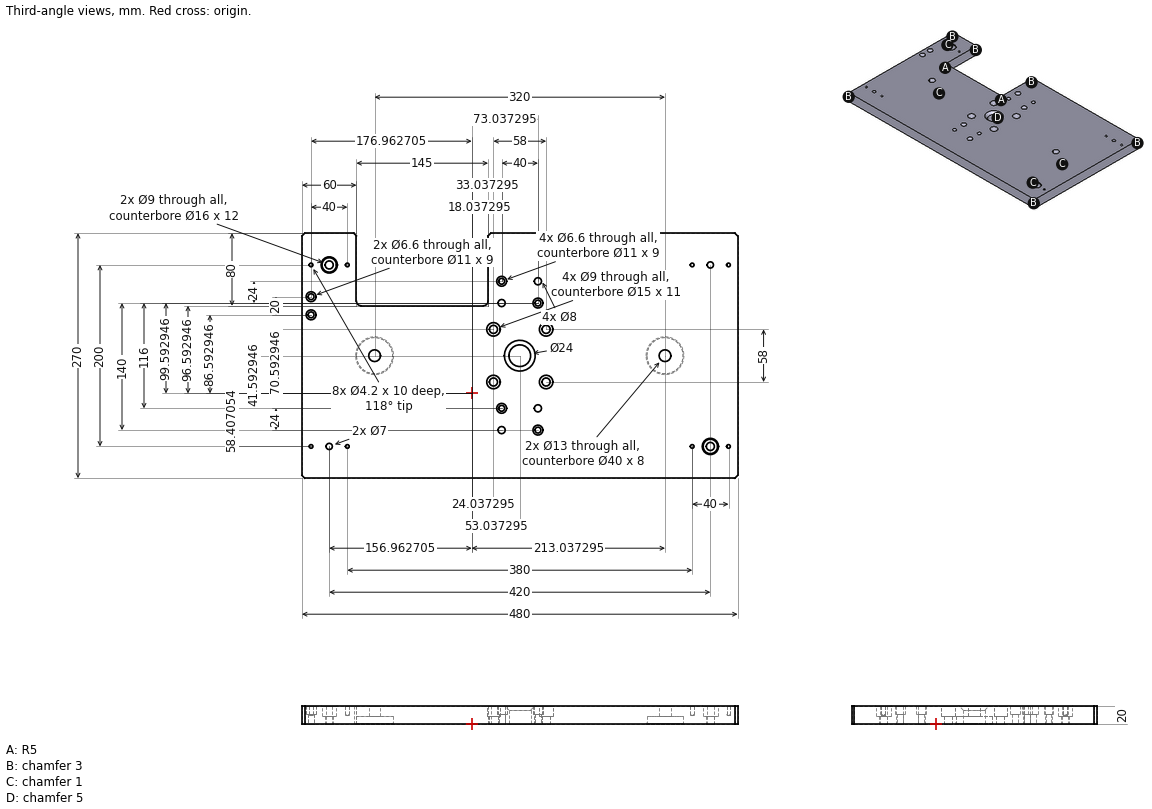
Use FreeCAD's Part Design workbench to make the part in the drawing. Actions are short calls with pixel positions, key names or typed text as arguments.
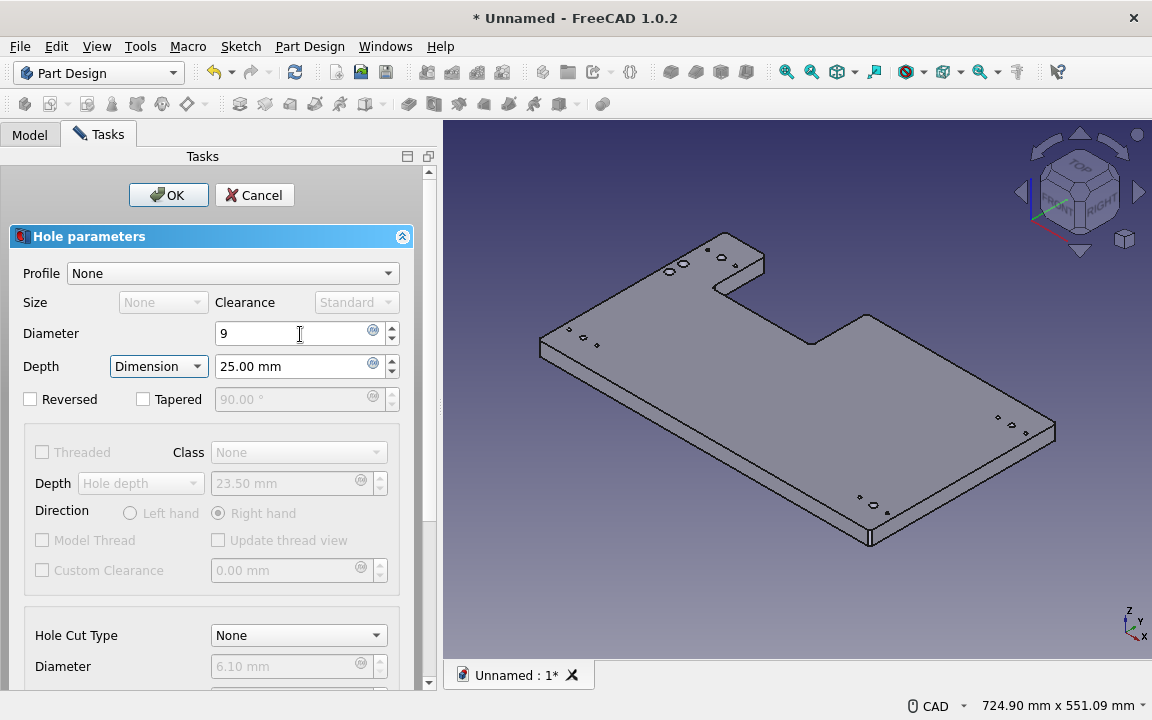
click(160, 366)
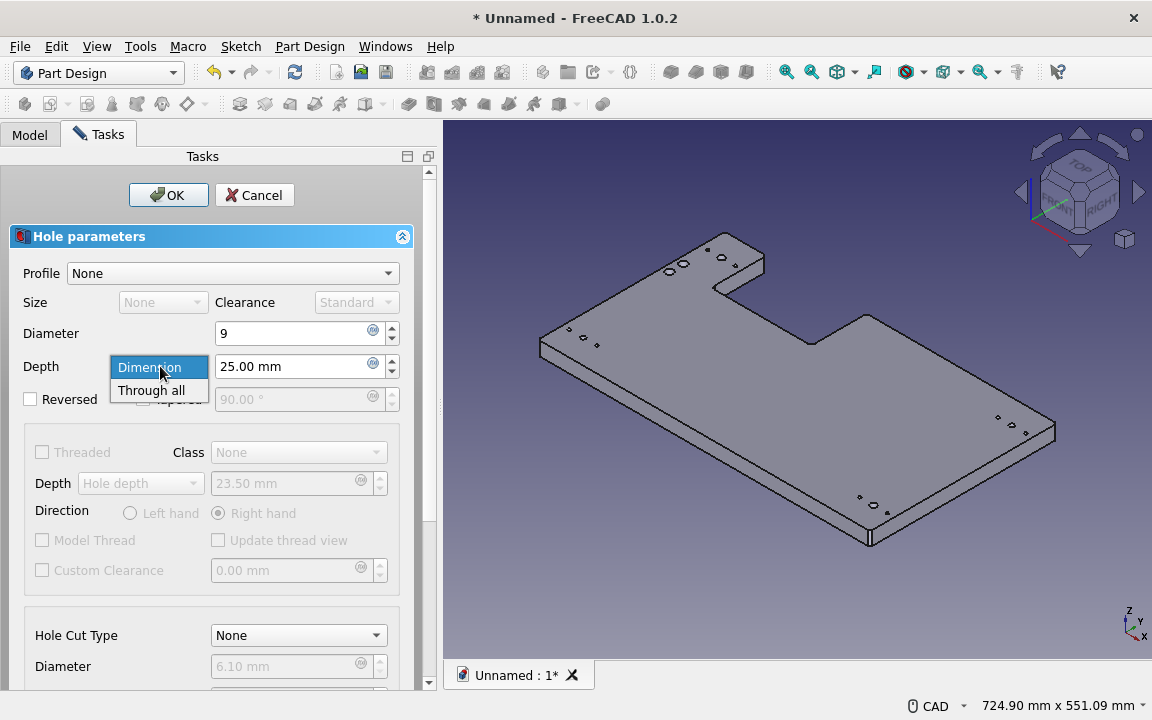
click(158, 390)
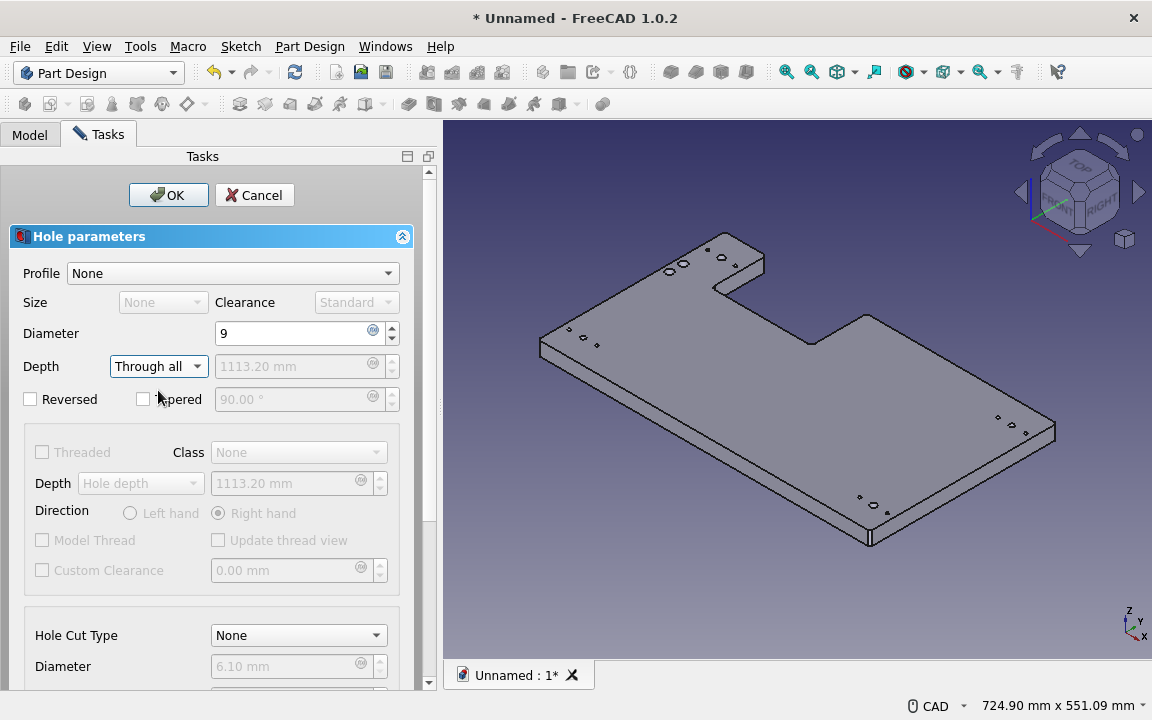
click(300, 636)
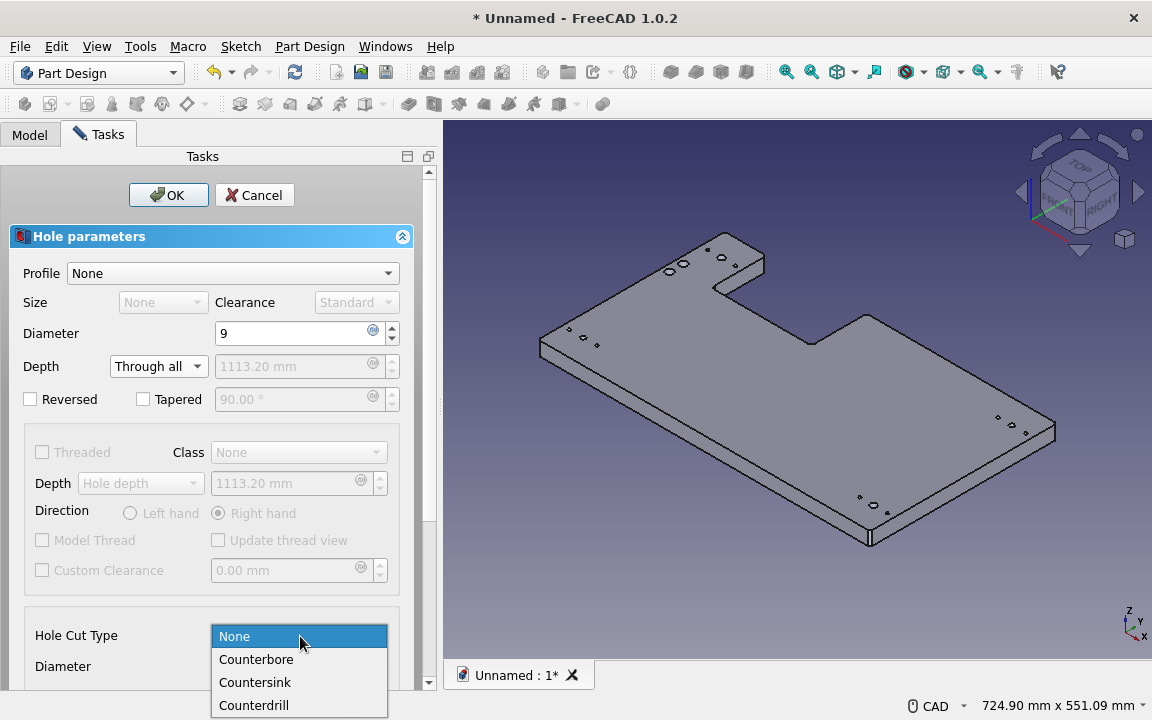
click(298, 660)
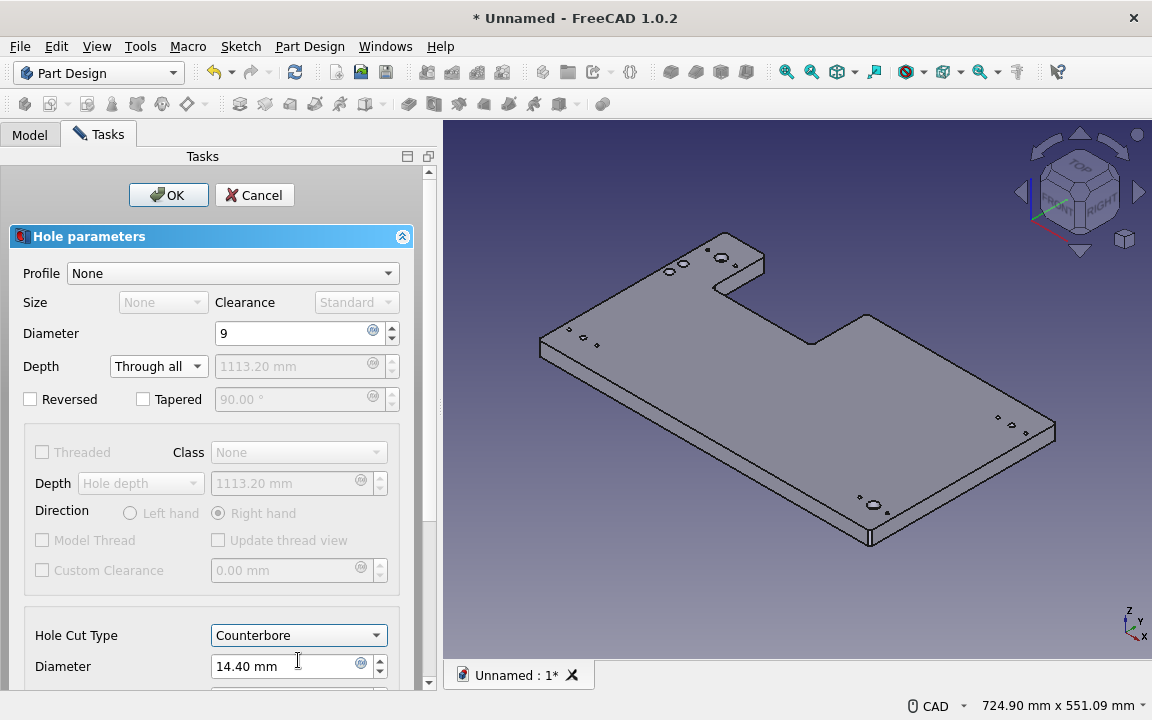
triple_click(292, 666)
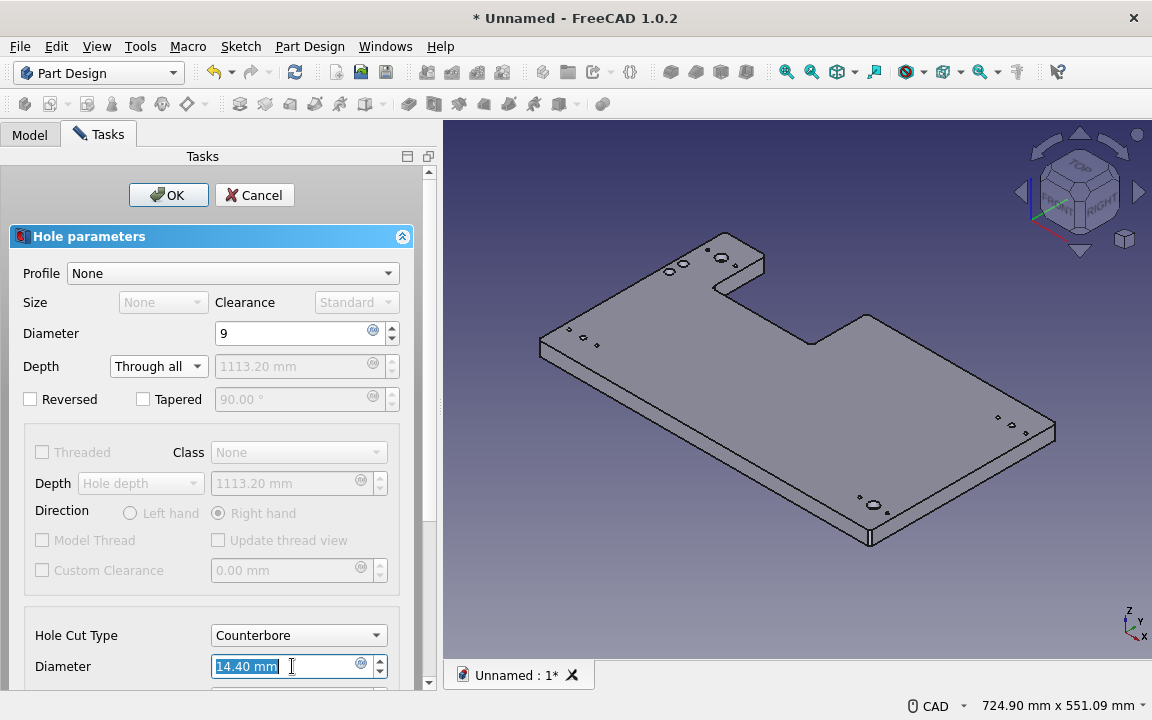
text(16)
key(Tab)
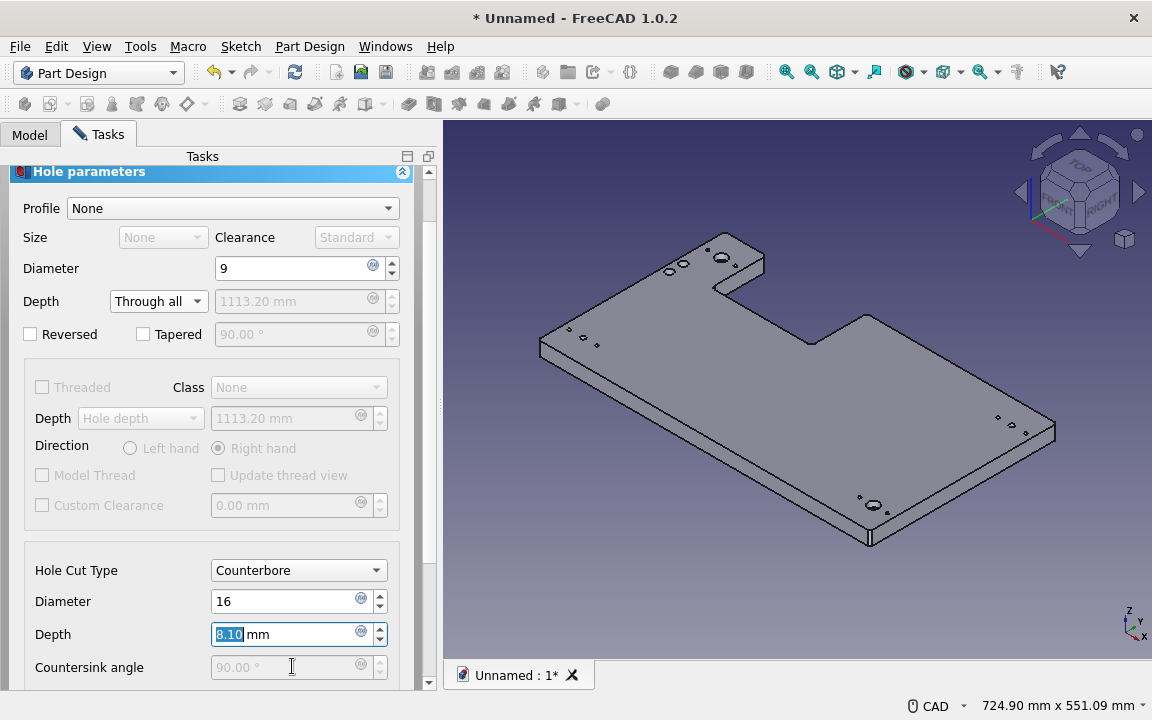
text(12)
key(Tab)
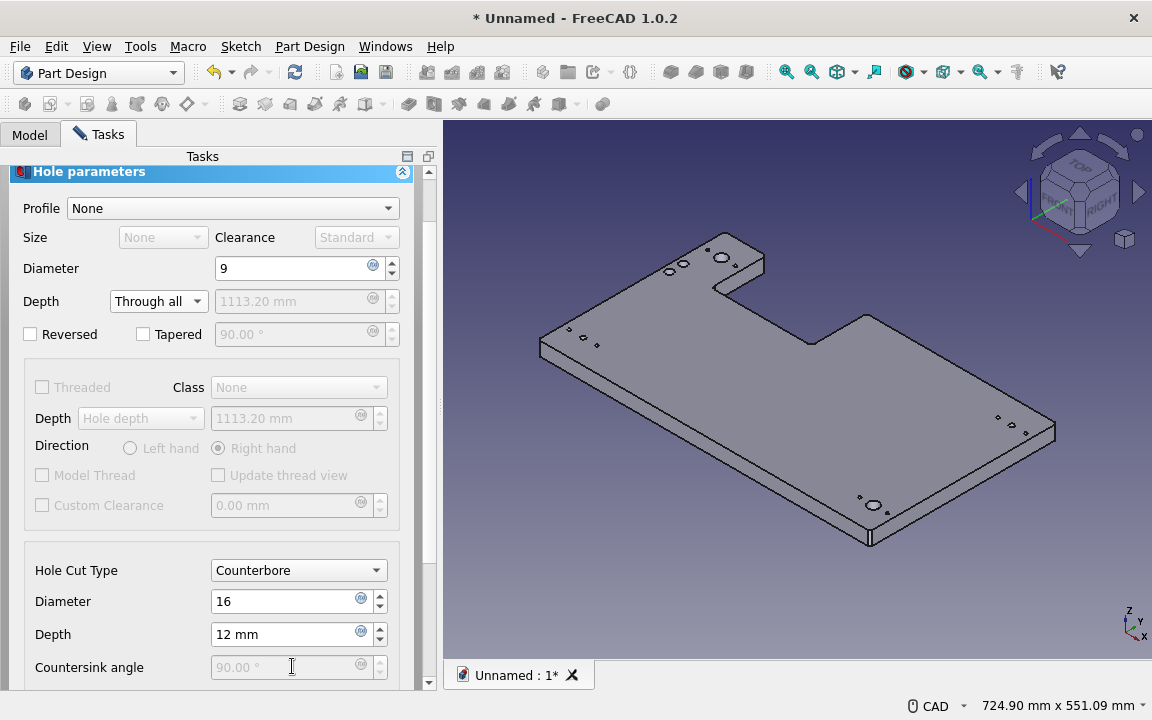
scroll(429, 428, up, 2)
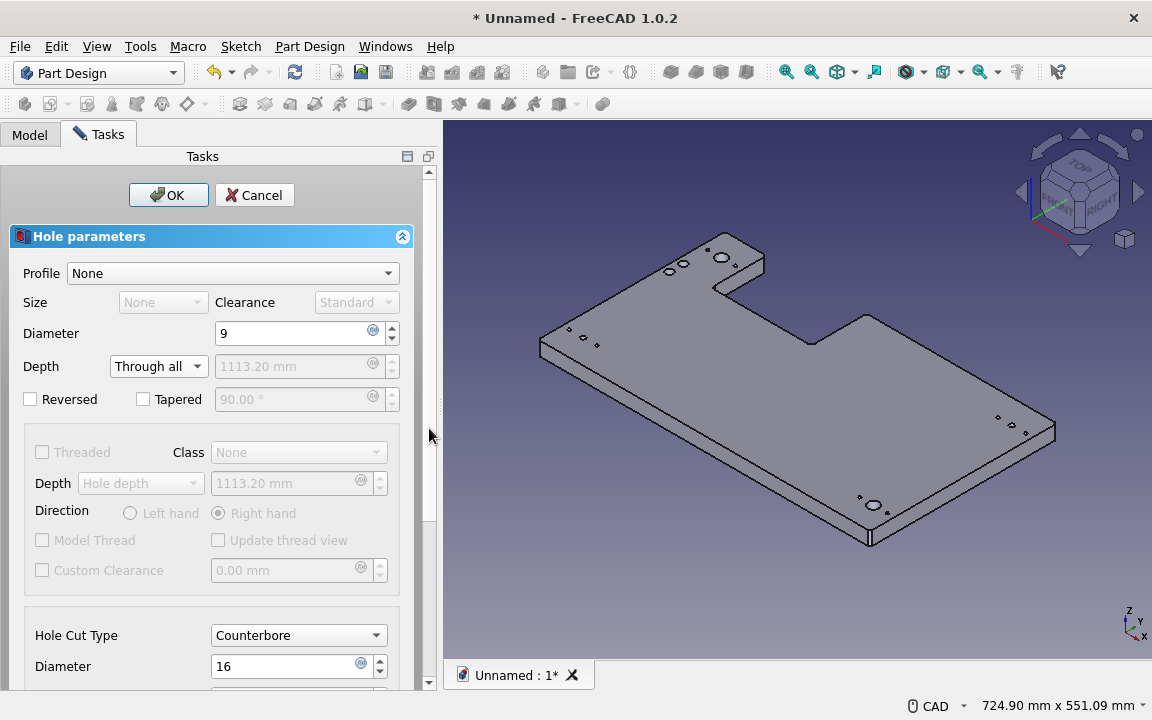
click(169, 195)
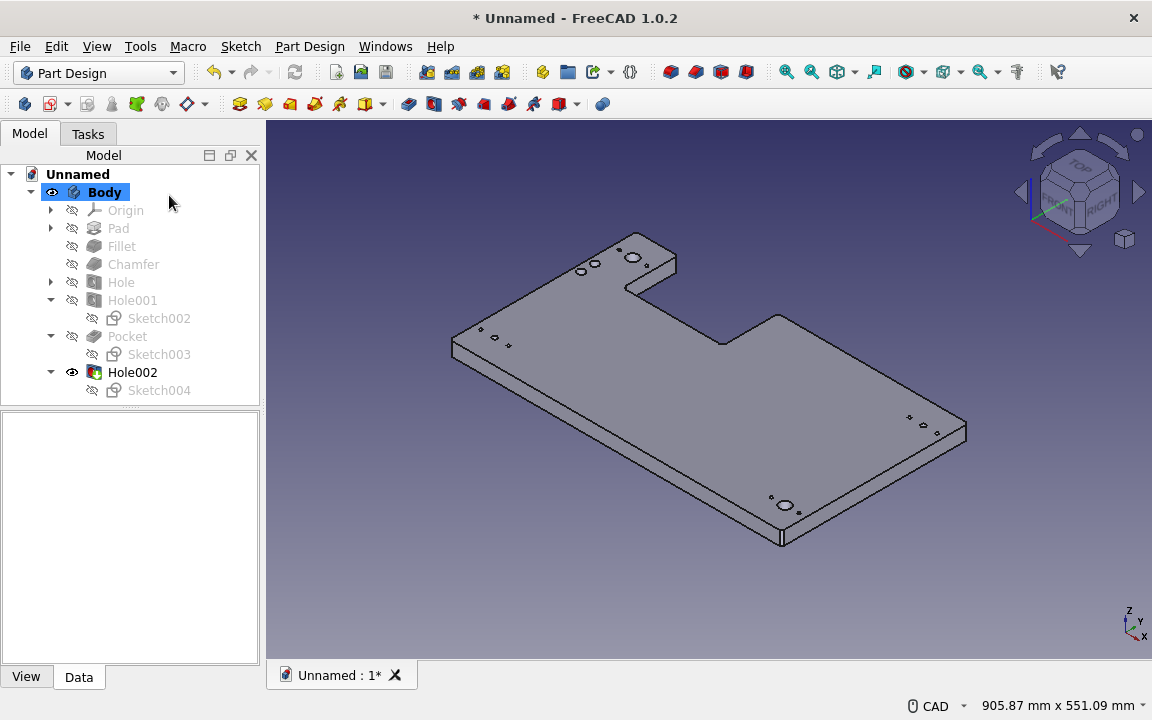
click(756, 408)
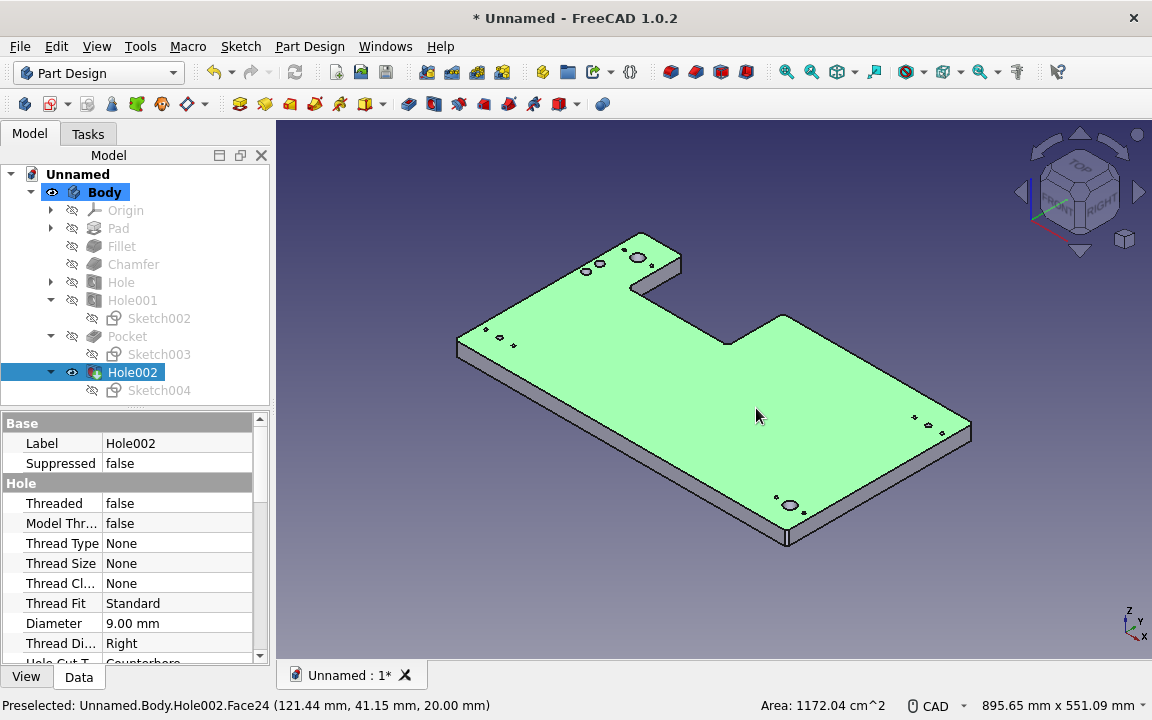
click(50, 104)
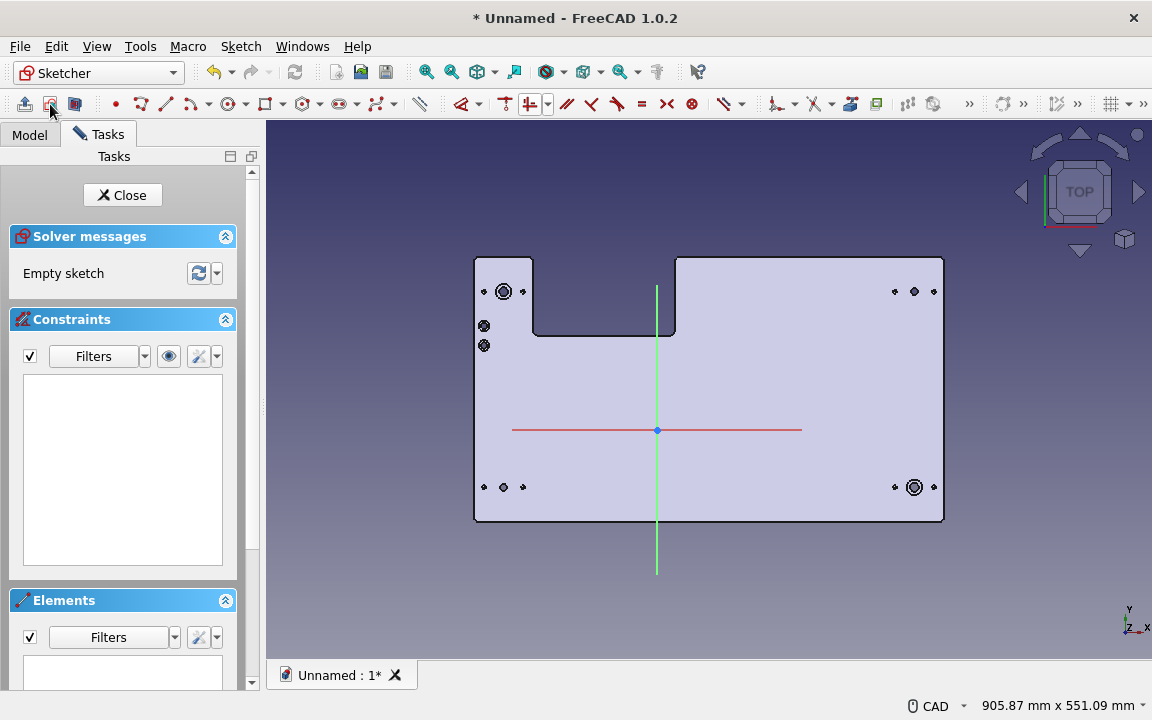
scroll(714, 394, up, 8)